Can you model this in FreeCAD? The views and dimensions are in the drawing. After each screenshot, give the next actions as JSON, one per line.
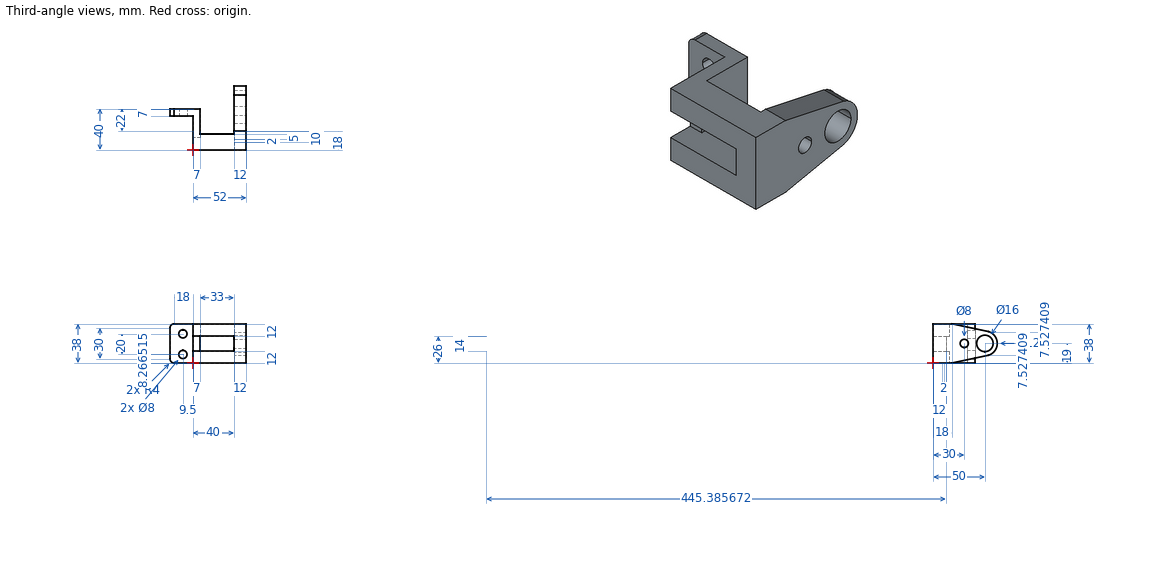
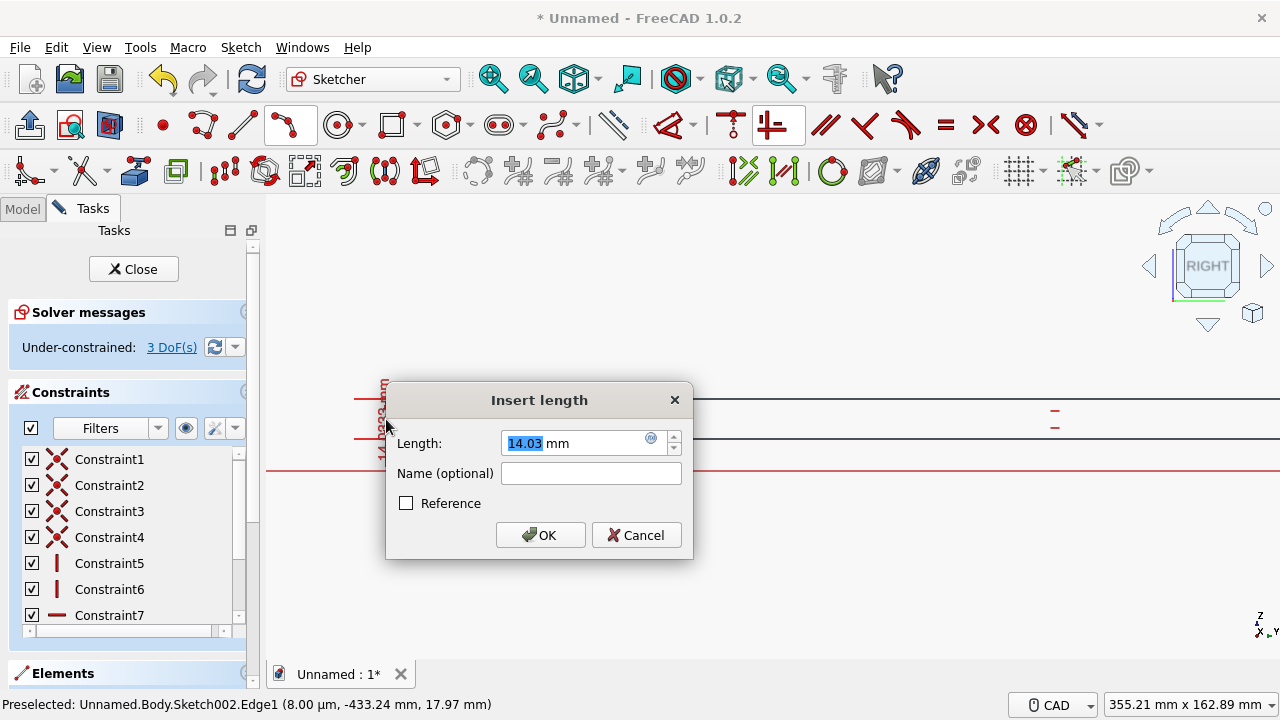
{"action": "type", "text": "14"}
{"action": "key", "text": "Return"}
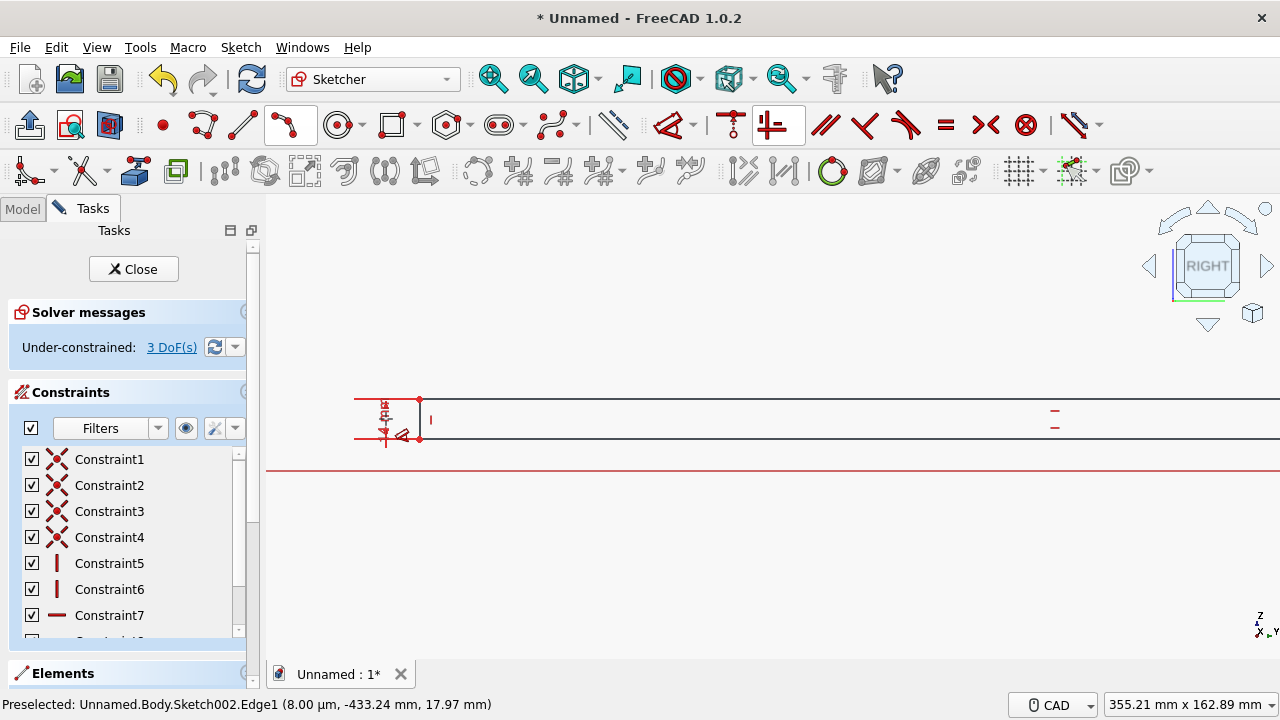
{"action": "left_click", "coordinate": [420, 399]}
{"action": "left_click", "coordinate": [386, 452]}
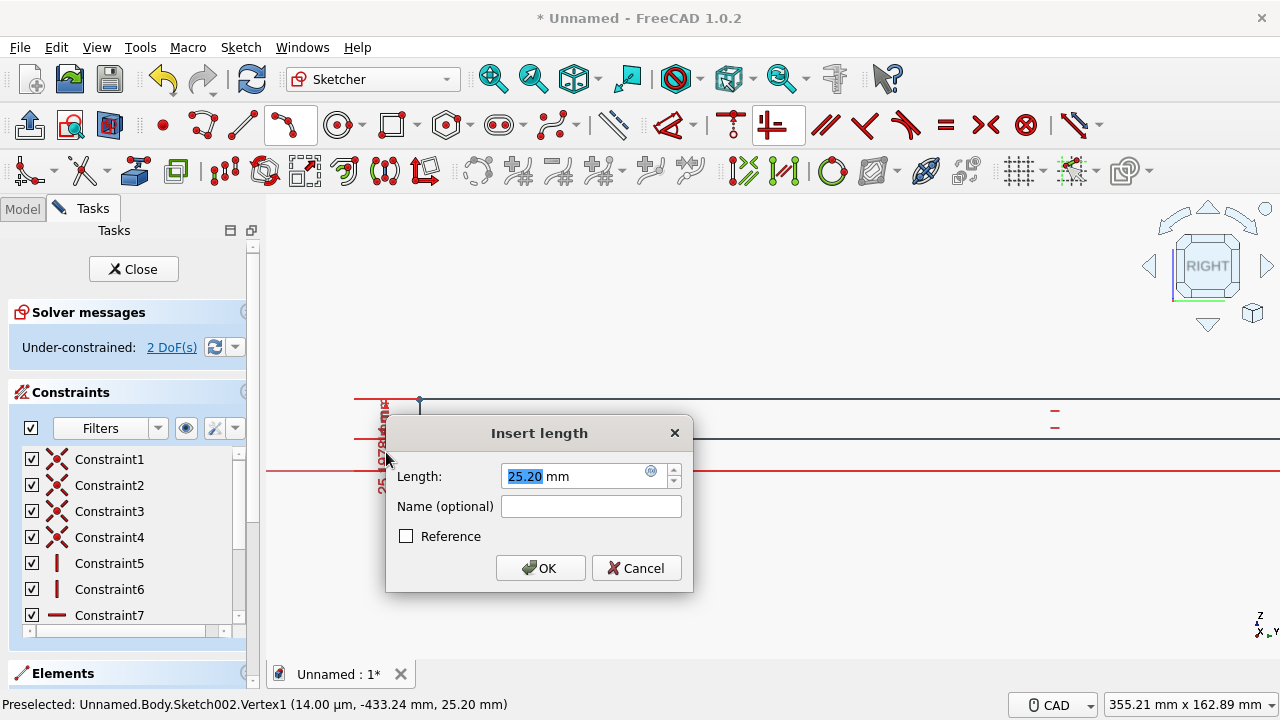
{"action": "type", "text": "26"}
{"action": "key", "text": "Return"}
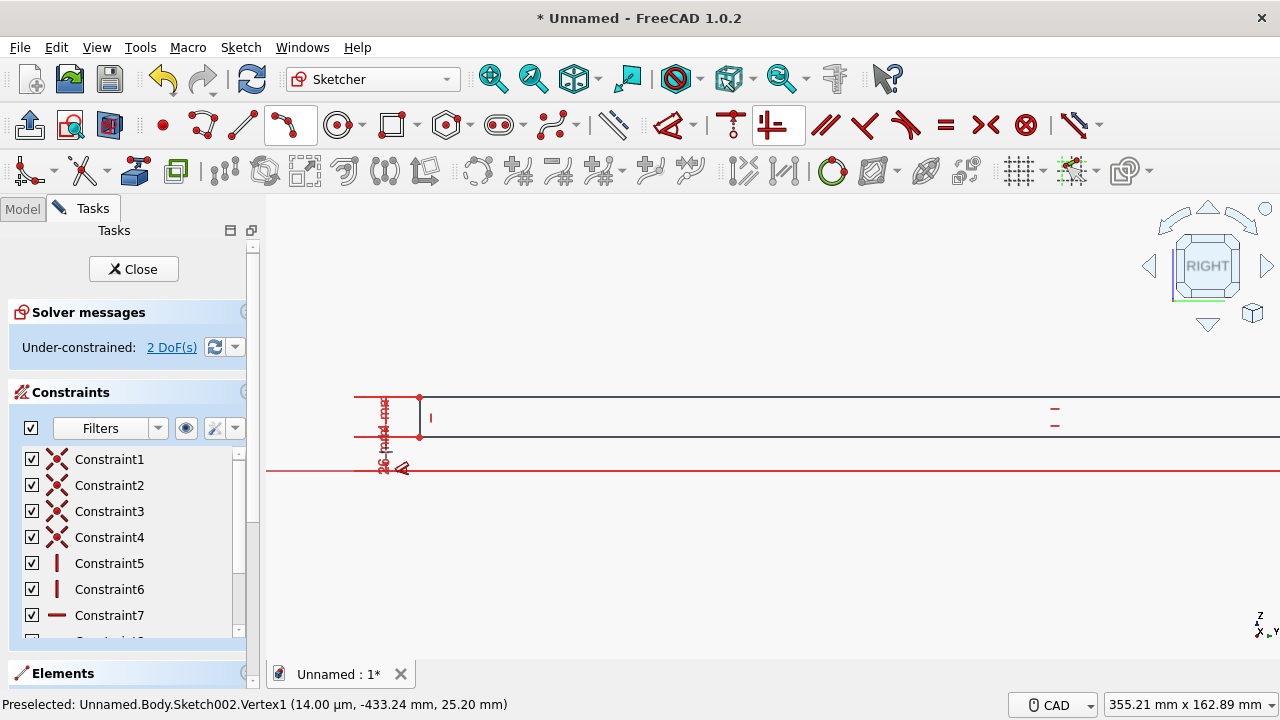
{"action": "scroll", "coordinate": [418, 420], "scroll_direction": "down", "scroll_amount": 4}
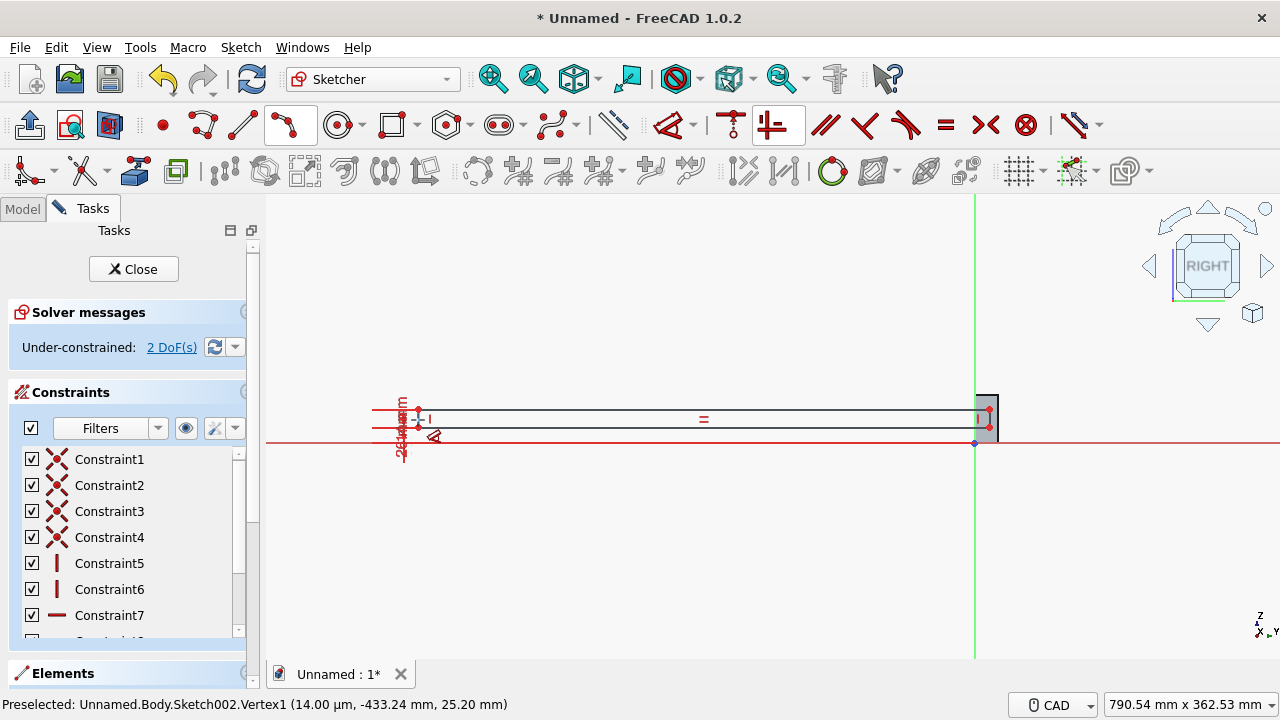
{"action": "scroll", "coordinate": [990, 428], "scroll_direction": "up", "scroll_amount": 5}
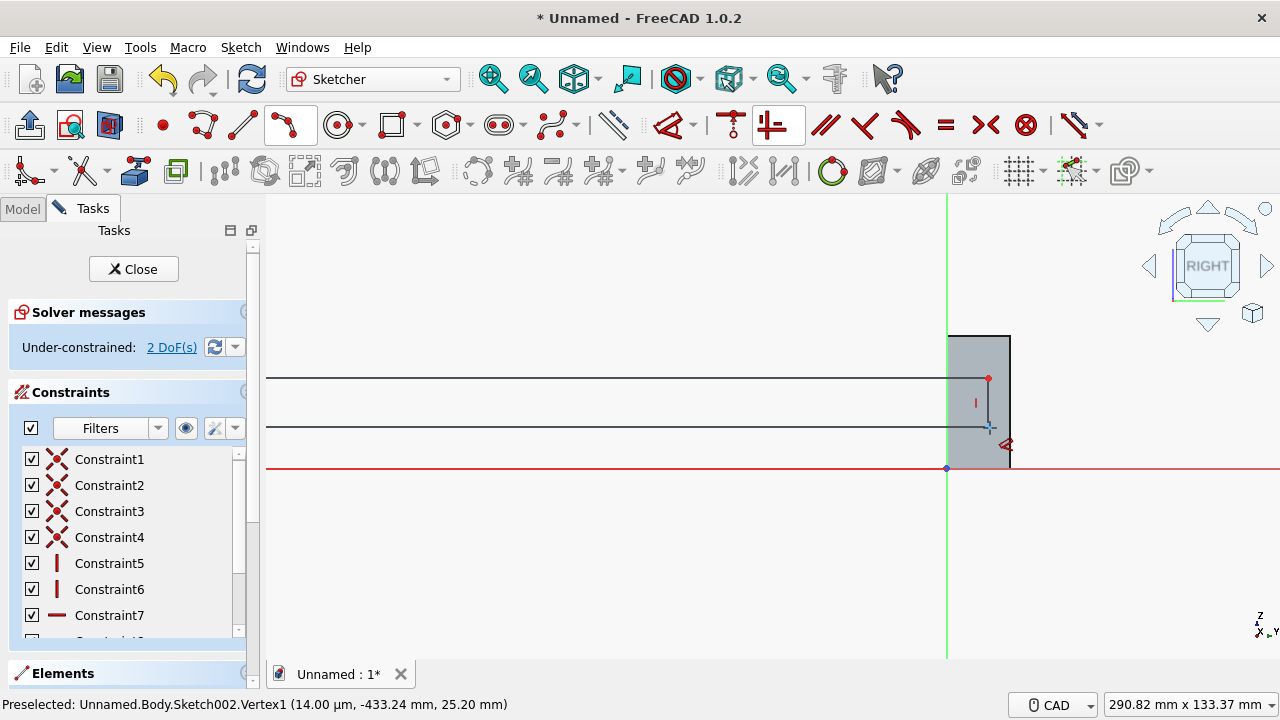
{"action": "left_click", "coordinate": [988, 427]}
{"action": "left_click", "coordinate": [968, 503]}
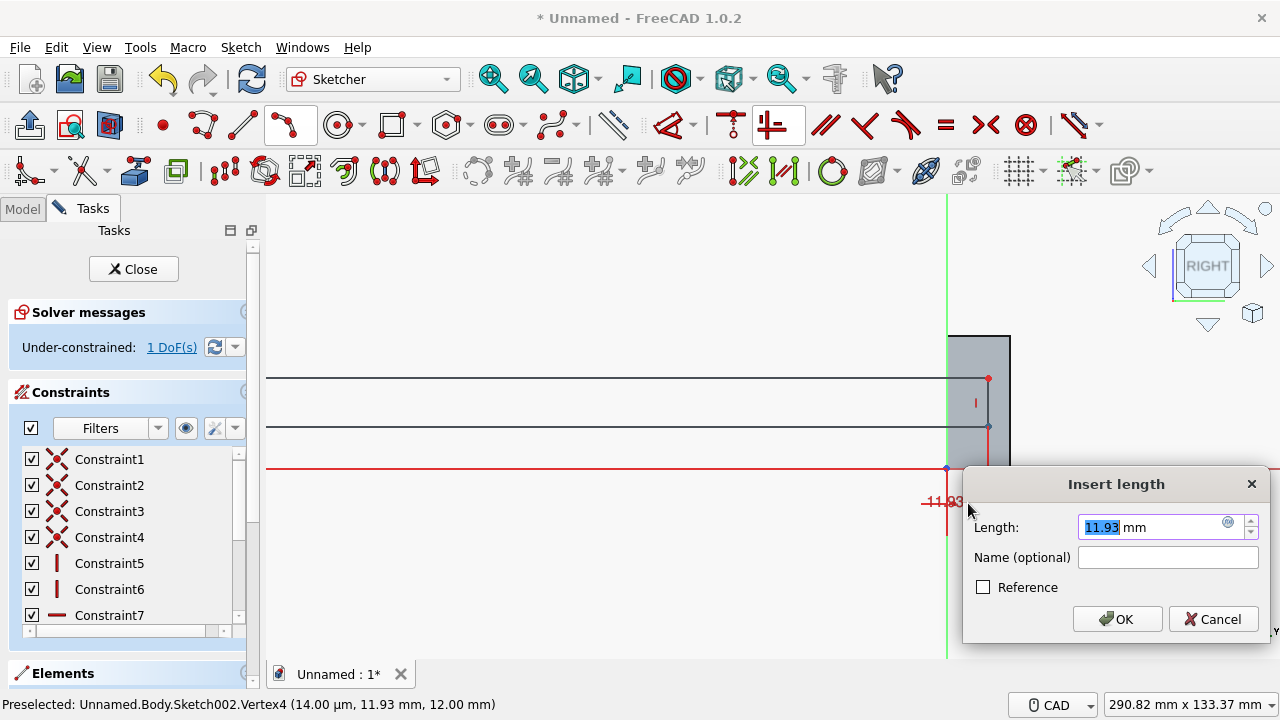
{"action": "type", "text": "12"}
{"action": "key", "text": "Return"}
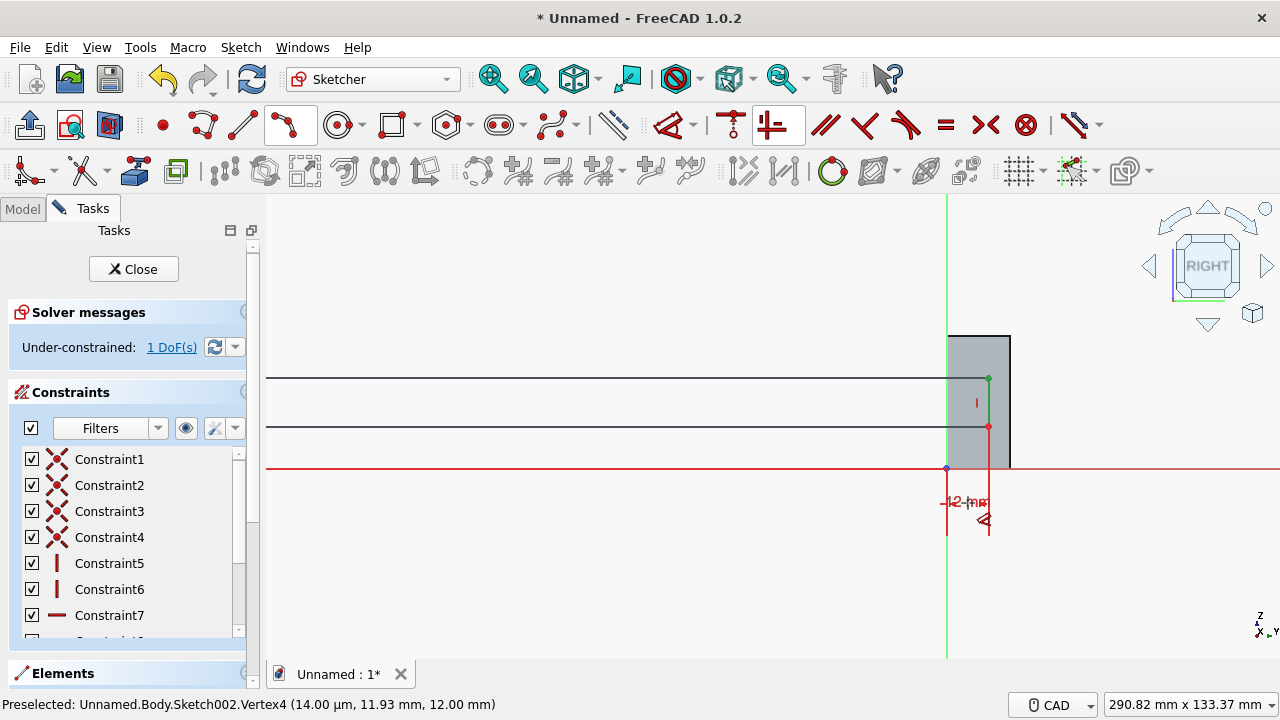
{"action": "left_click", "coordinate": [523, 427]}
{"action": "left_click", "coordinate": [641, 393]}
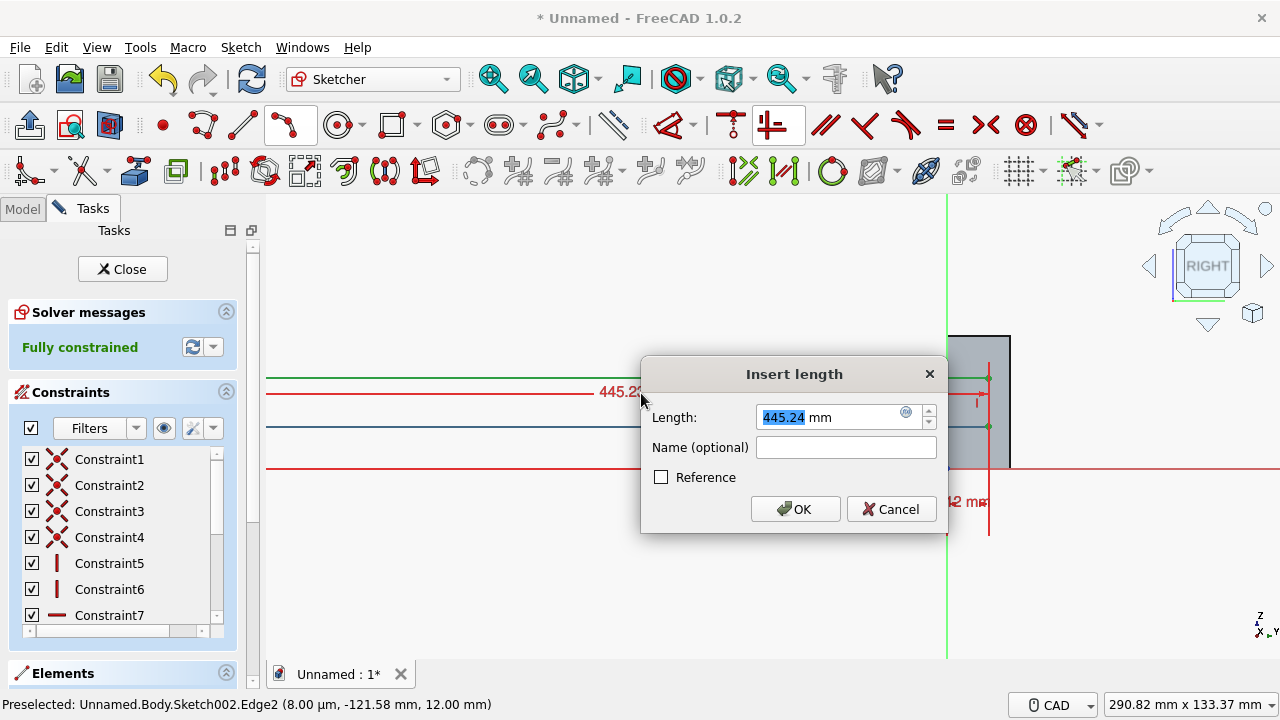
{"action": "type", "text": "445.385672"}
{"action": "key", "text": "Return"}
{"action": "key", "text": "Escape"}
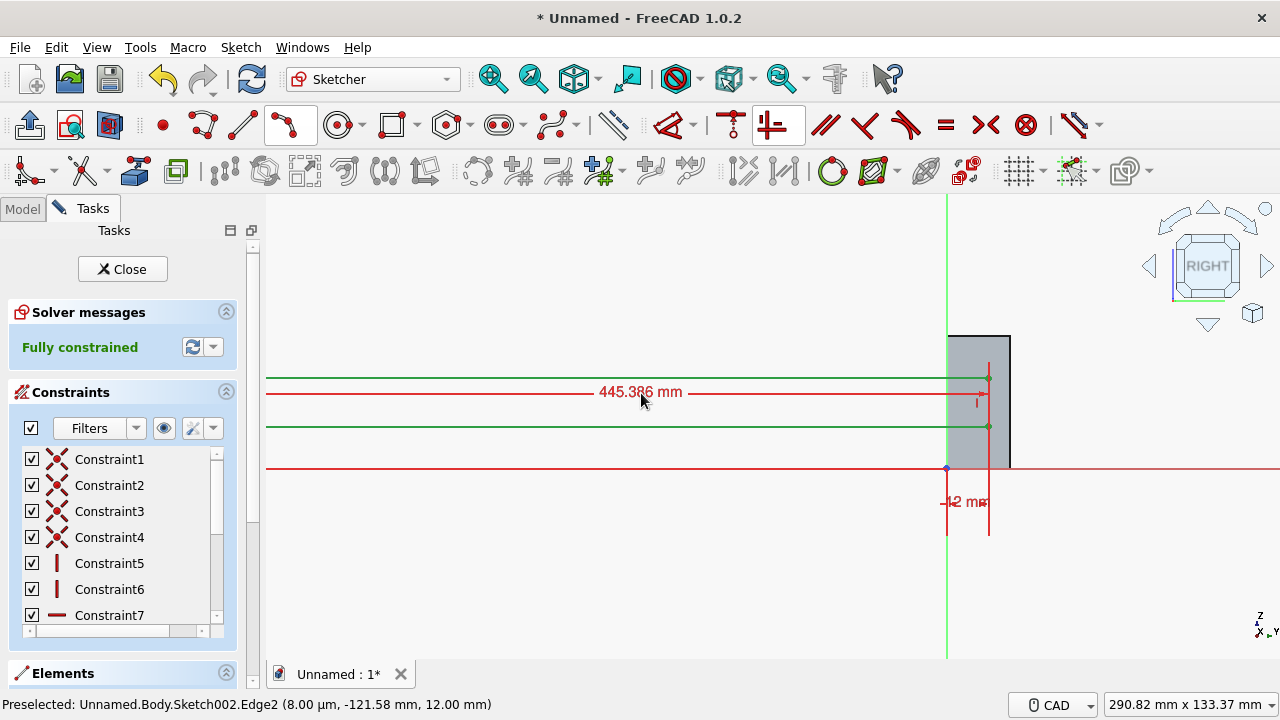
{"action": "left_click", "coordinate": [123, 269]}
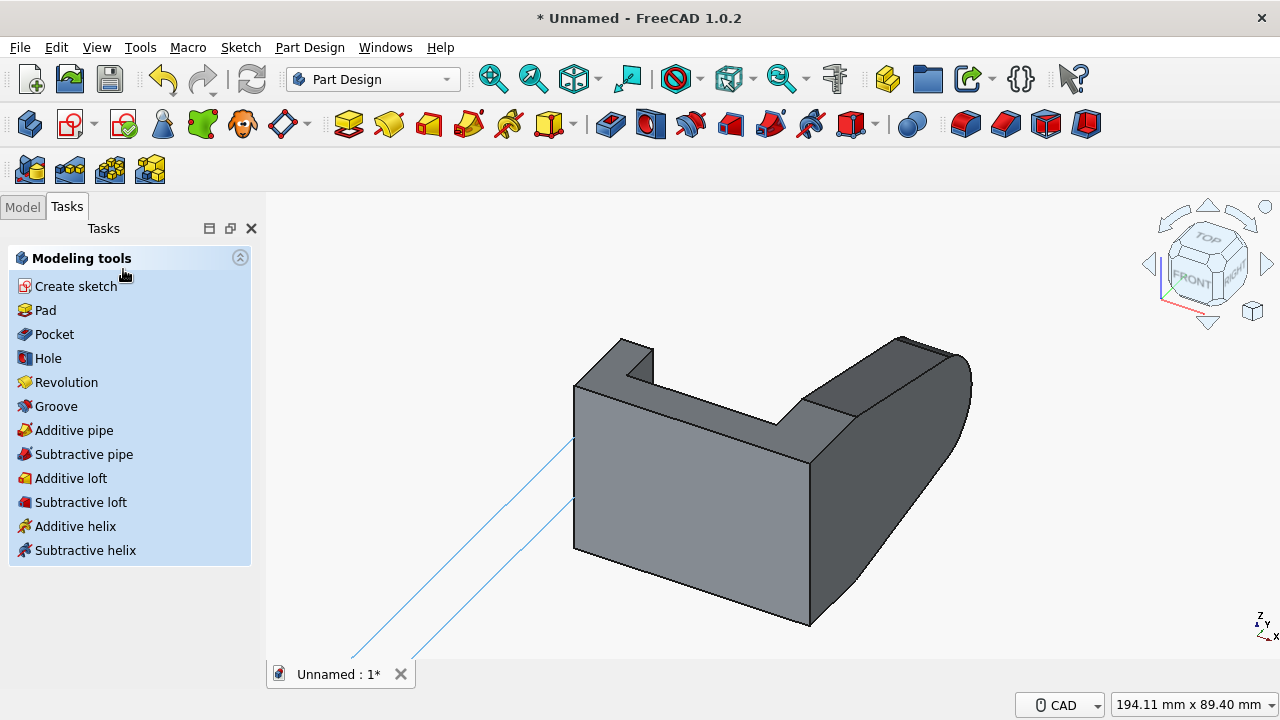
{"action": "left_click", "coordinate": [612, 124]}